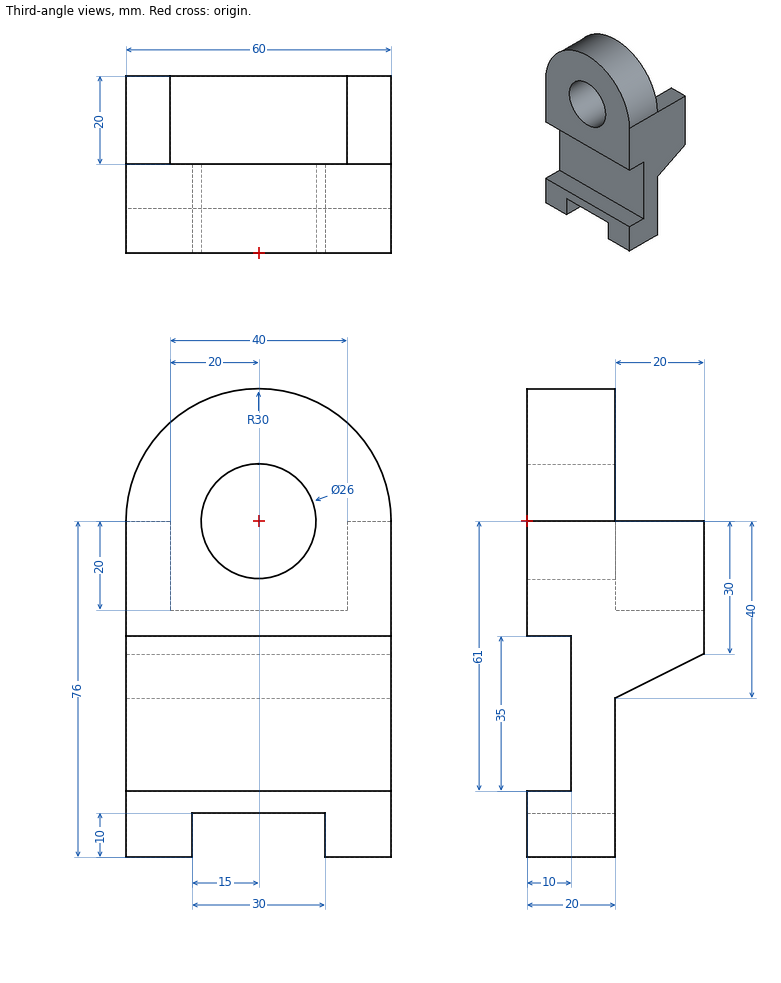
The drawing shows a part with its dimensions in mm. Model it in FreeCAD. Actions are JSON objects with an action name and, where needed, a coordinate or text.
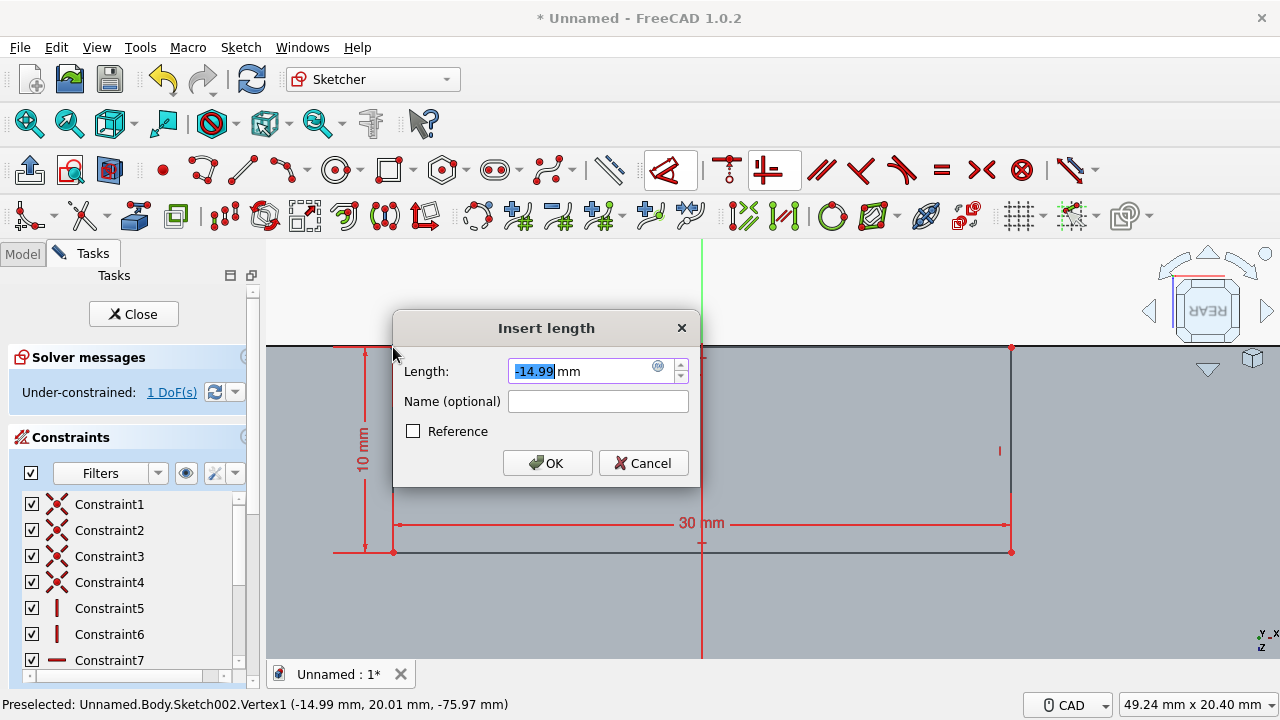
{"action": "type", "text": "-15"}
{"action": "key", "text": "Return"}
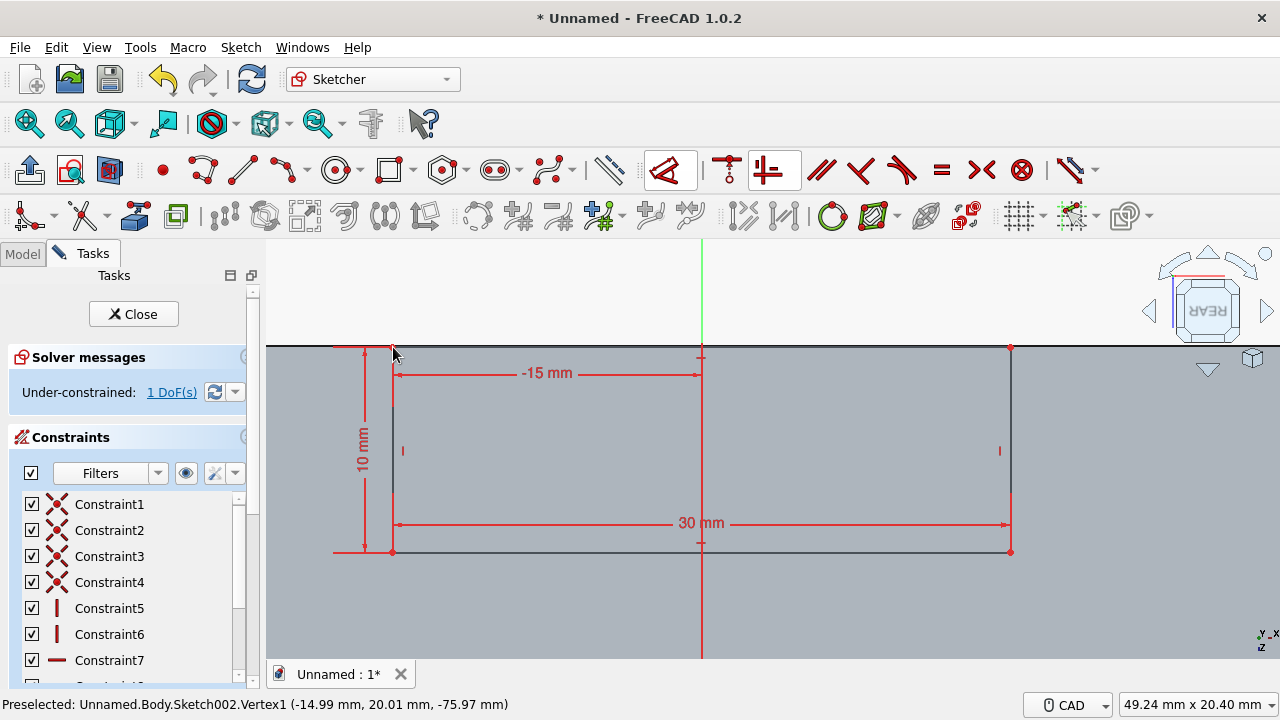
{"action": "left_click", "coordinate": [393, 347]}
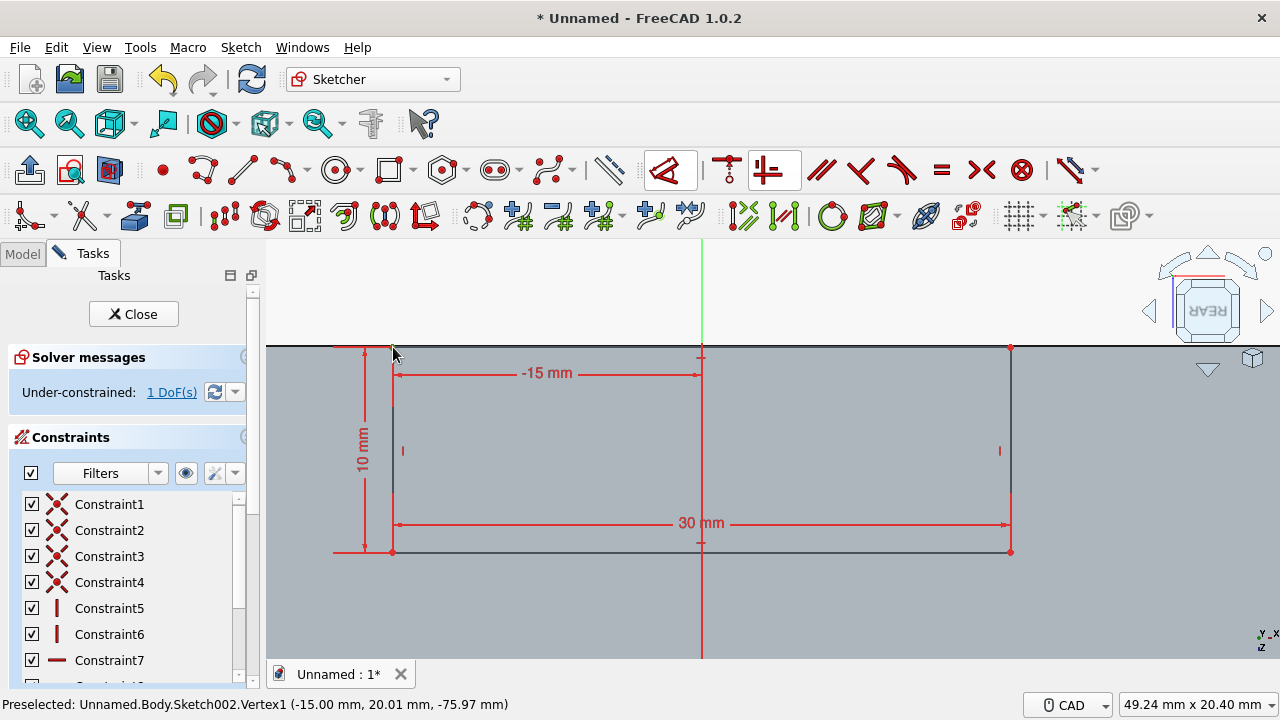
{"action": "key", "text": "i"}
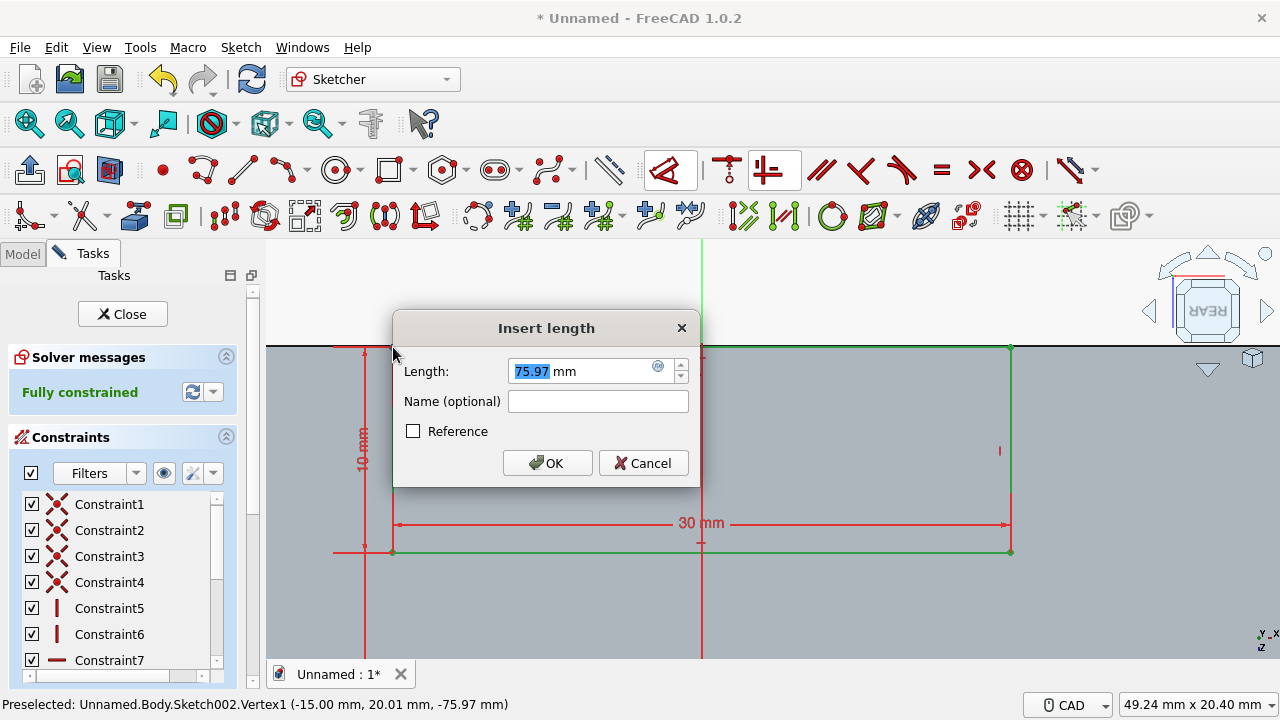
{"action": "type", "text": "76"}
{"action": "key", "text": "Return"}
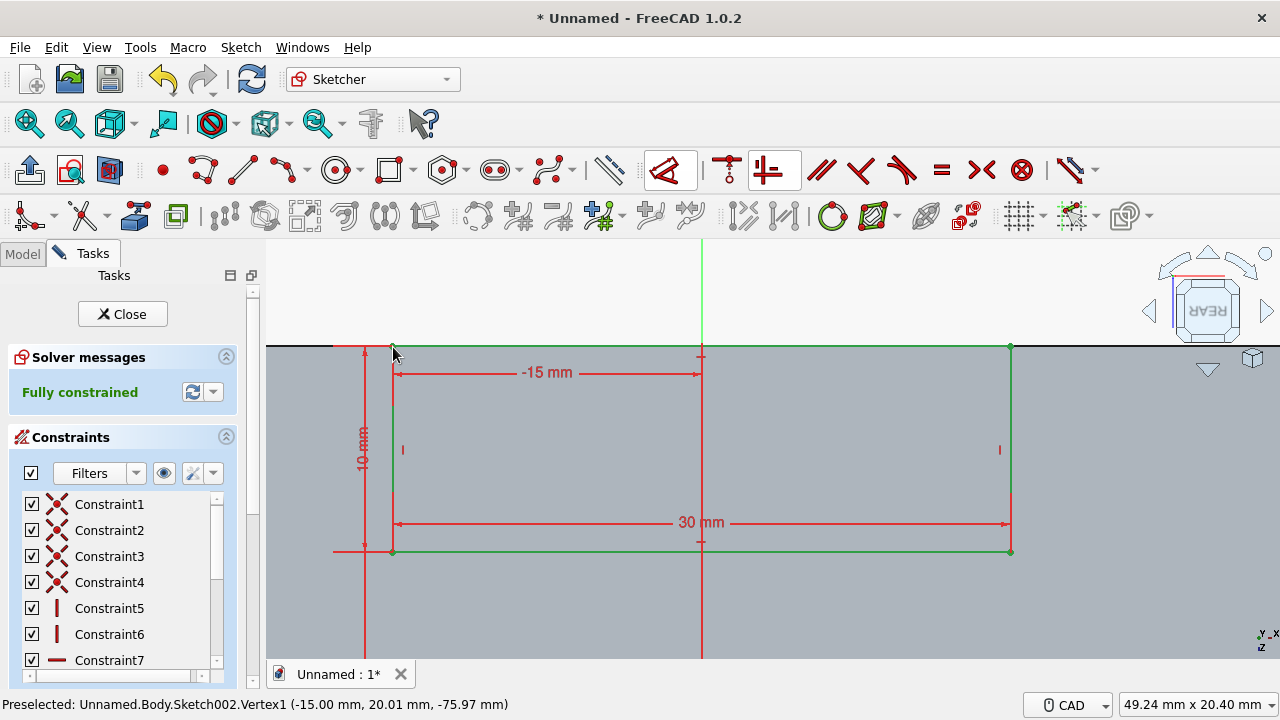
{"action": "left_click", "coordinate": [123, 314]}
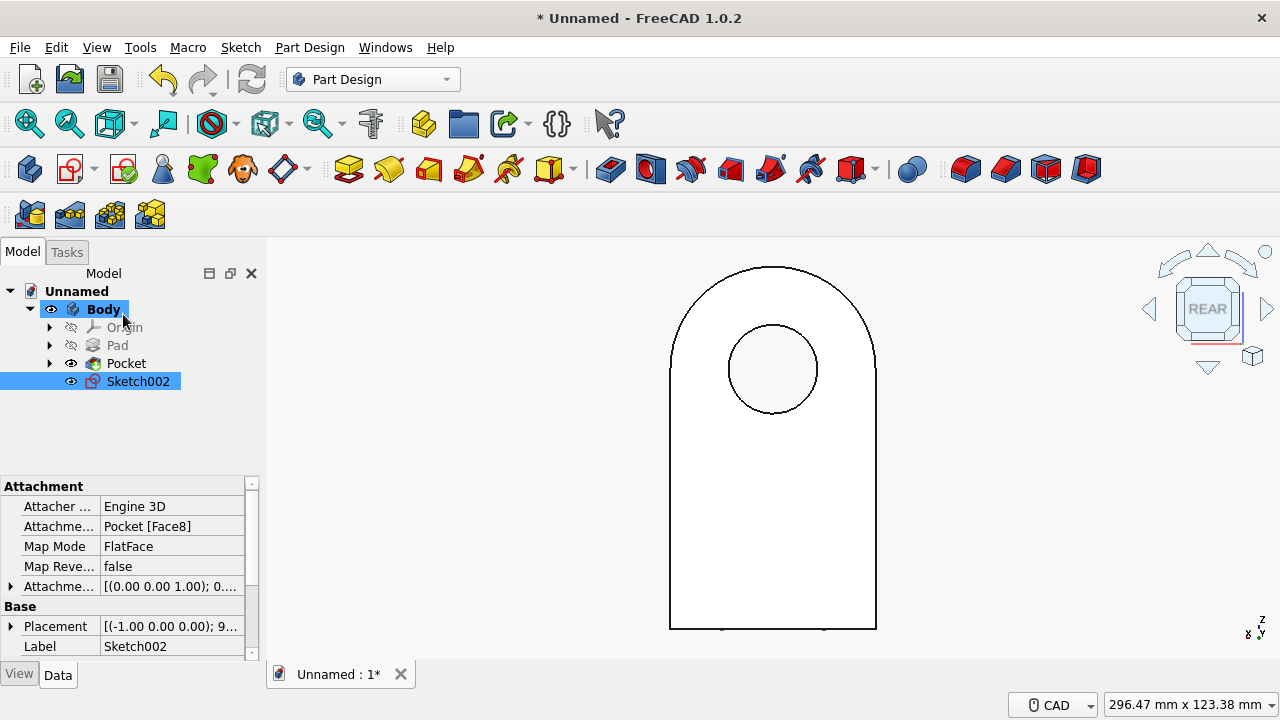
{"action": "left_click", "coordinate": [612, 170]}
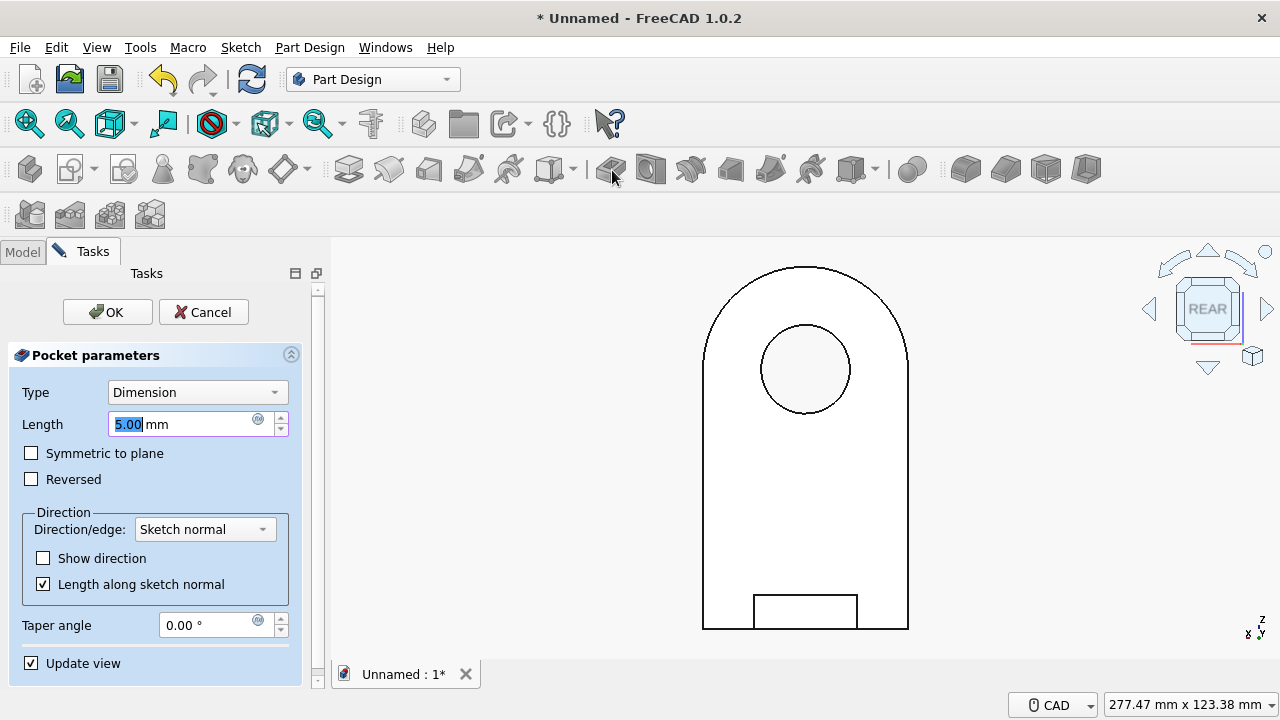
{"action": "left_click", "coordinate": [198, 392]}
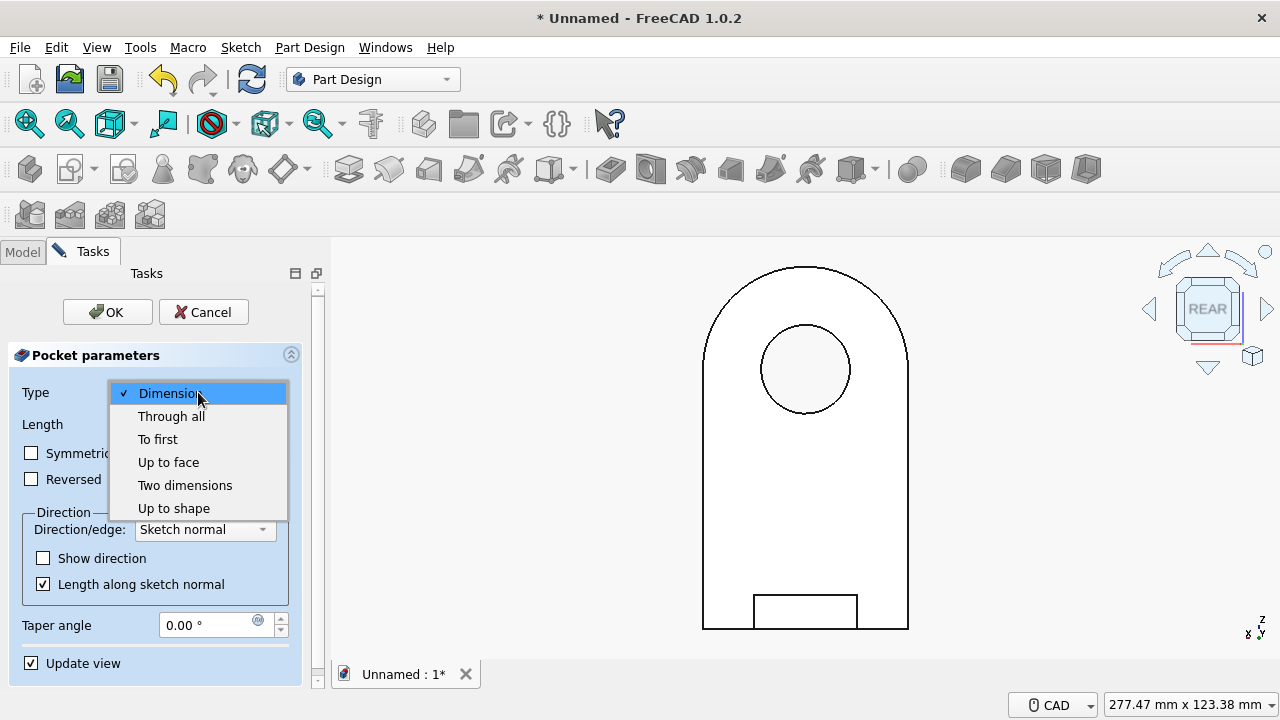
{"action": "left_click", "coordinate": [198, 440]}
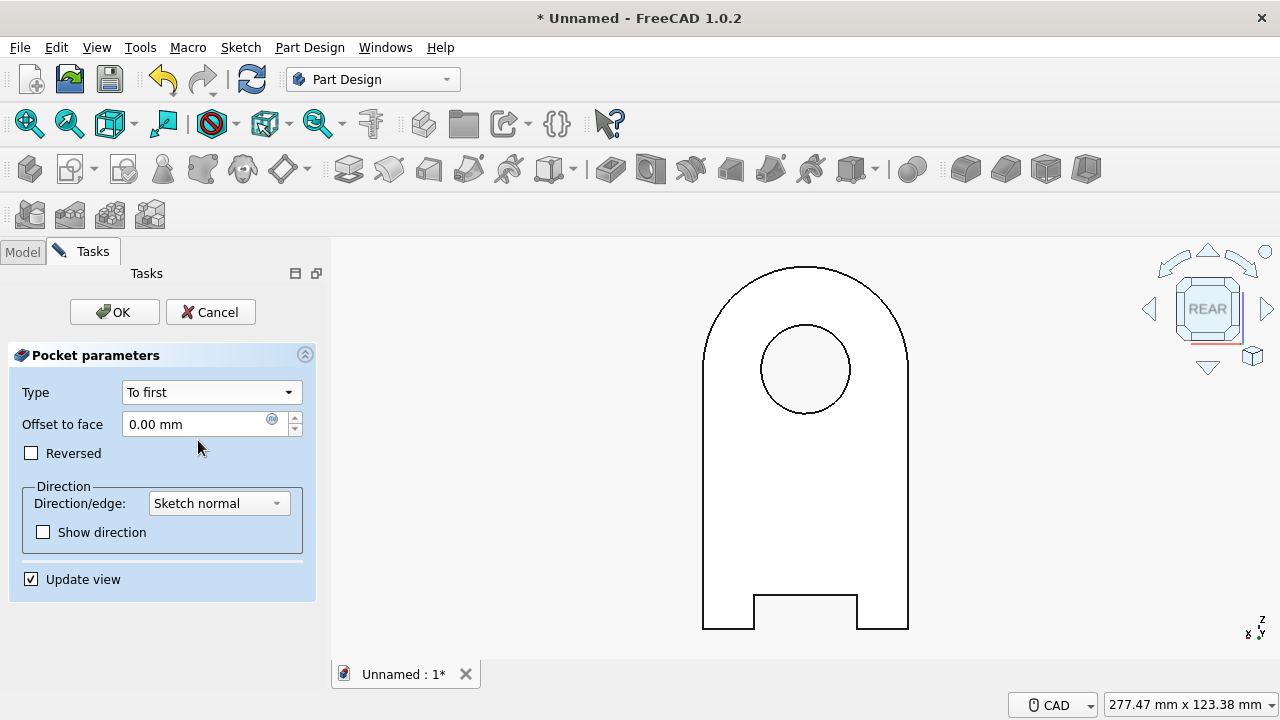
{"action": "left_click", "coordinate": [115, 312]}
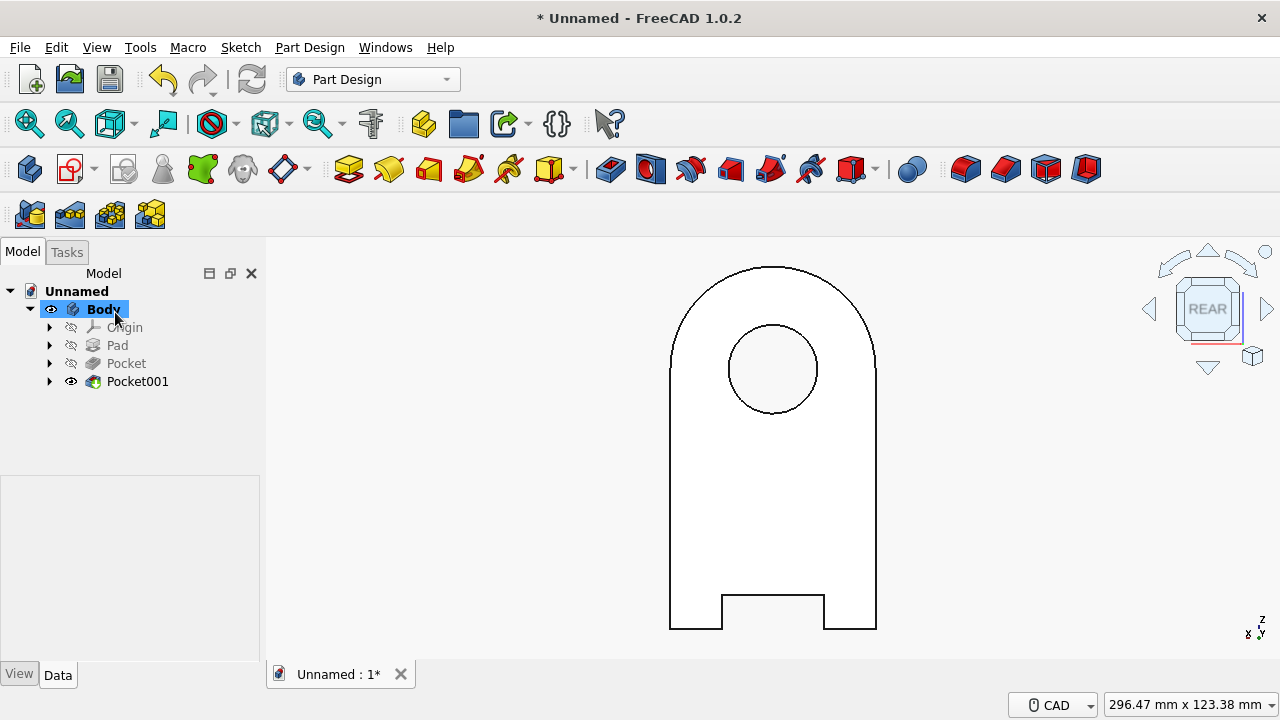
{"action": "left_click", "coordinate": [70, 170]}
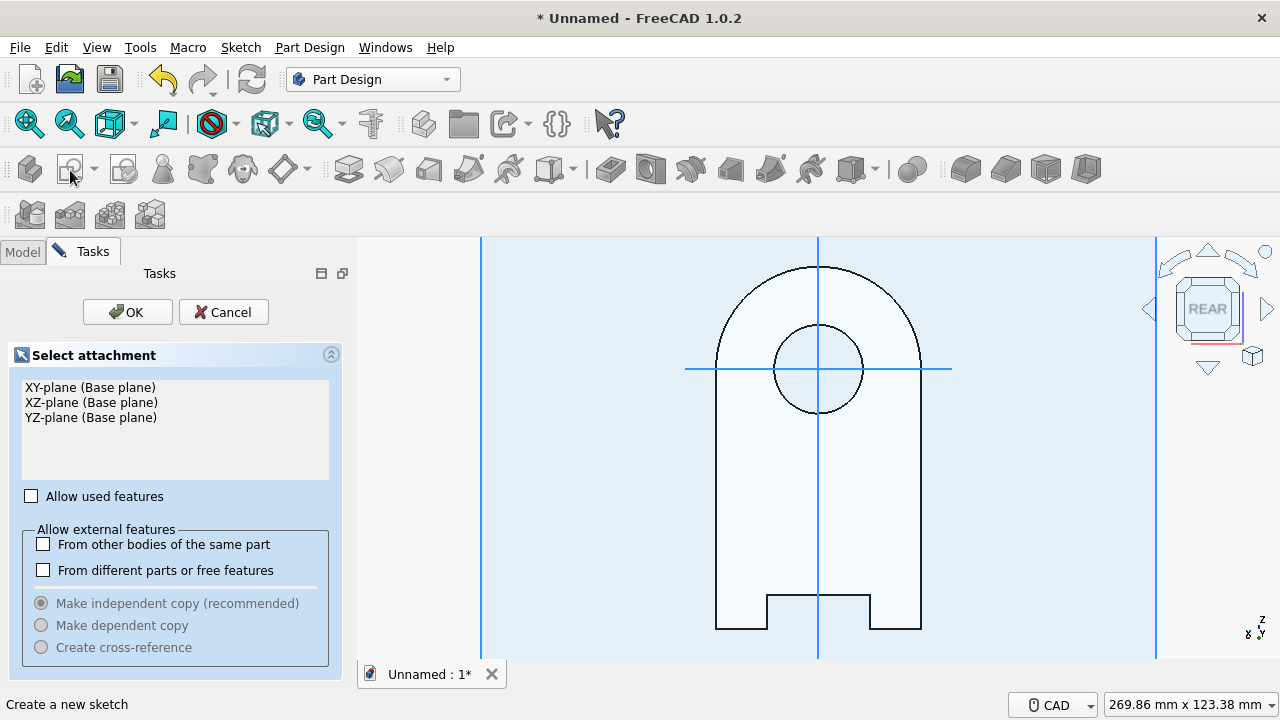
{"action": "left_click", "coordinate": [82, 418]}